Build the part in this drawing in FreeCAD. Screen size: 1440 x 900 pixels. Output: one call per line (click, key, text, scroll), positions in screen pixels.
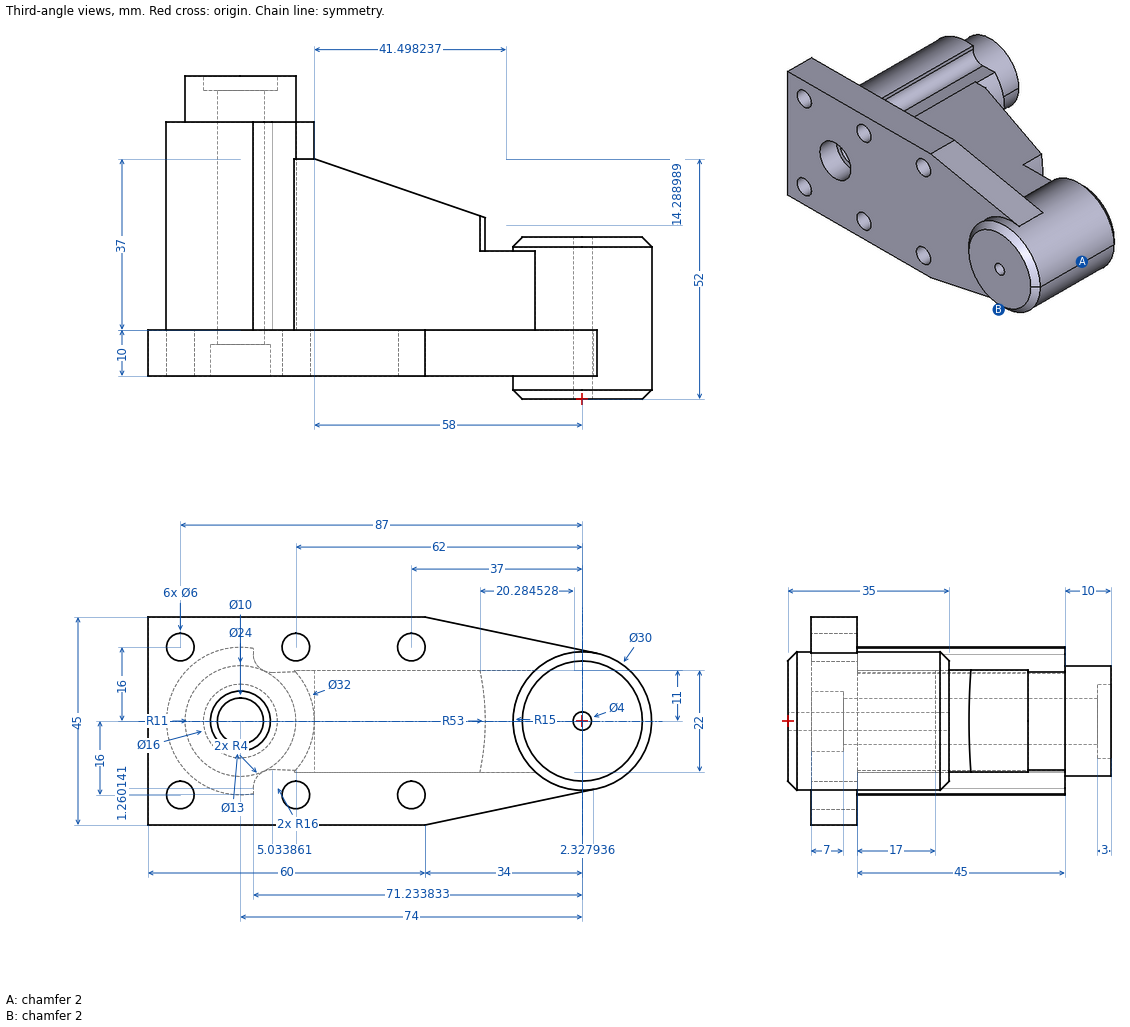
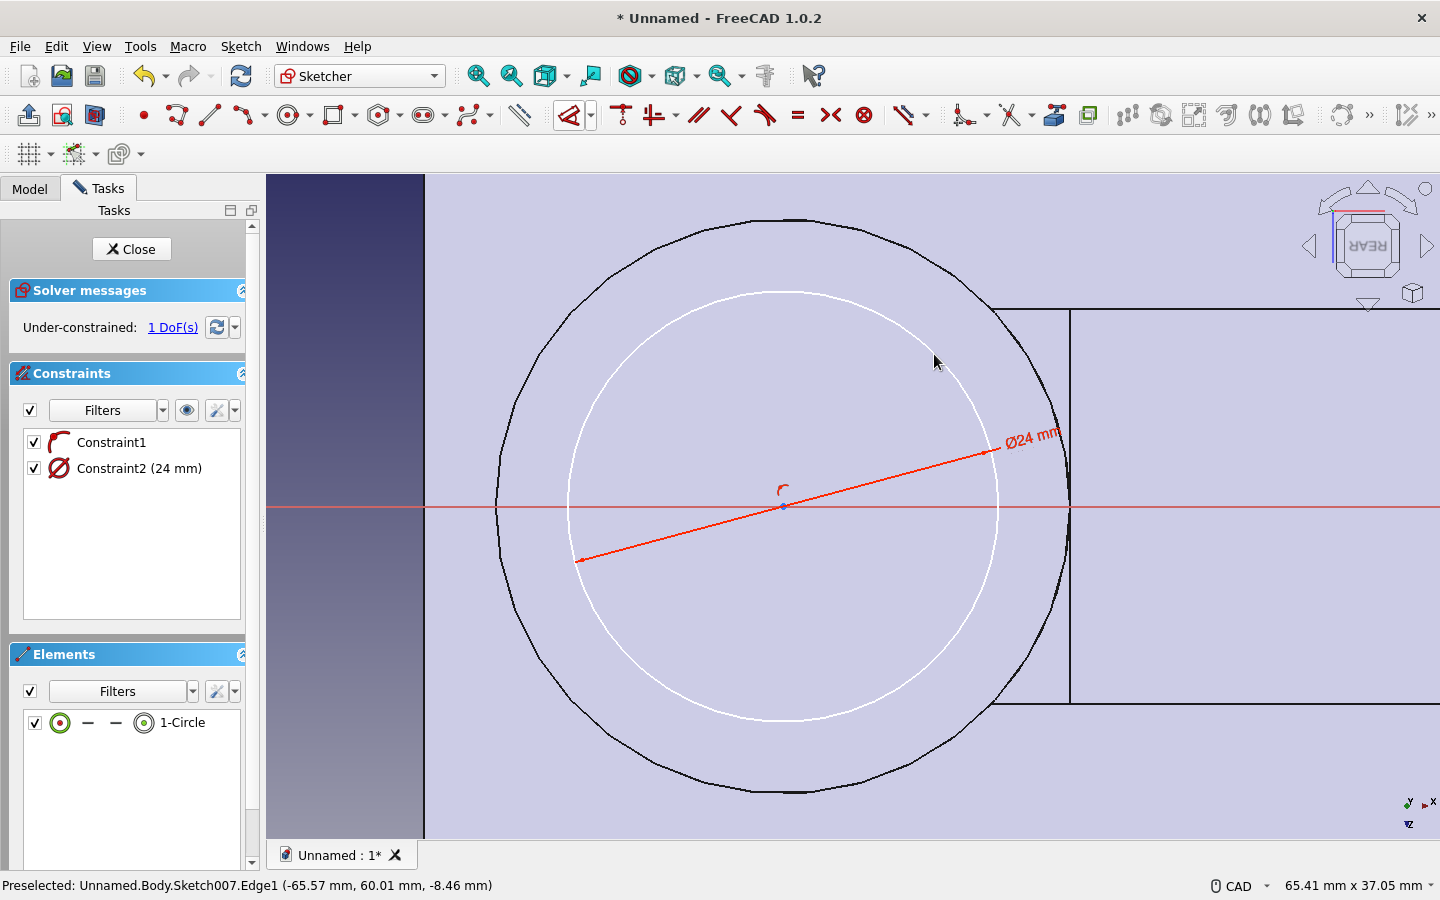
click(783, 506)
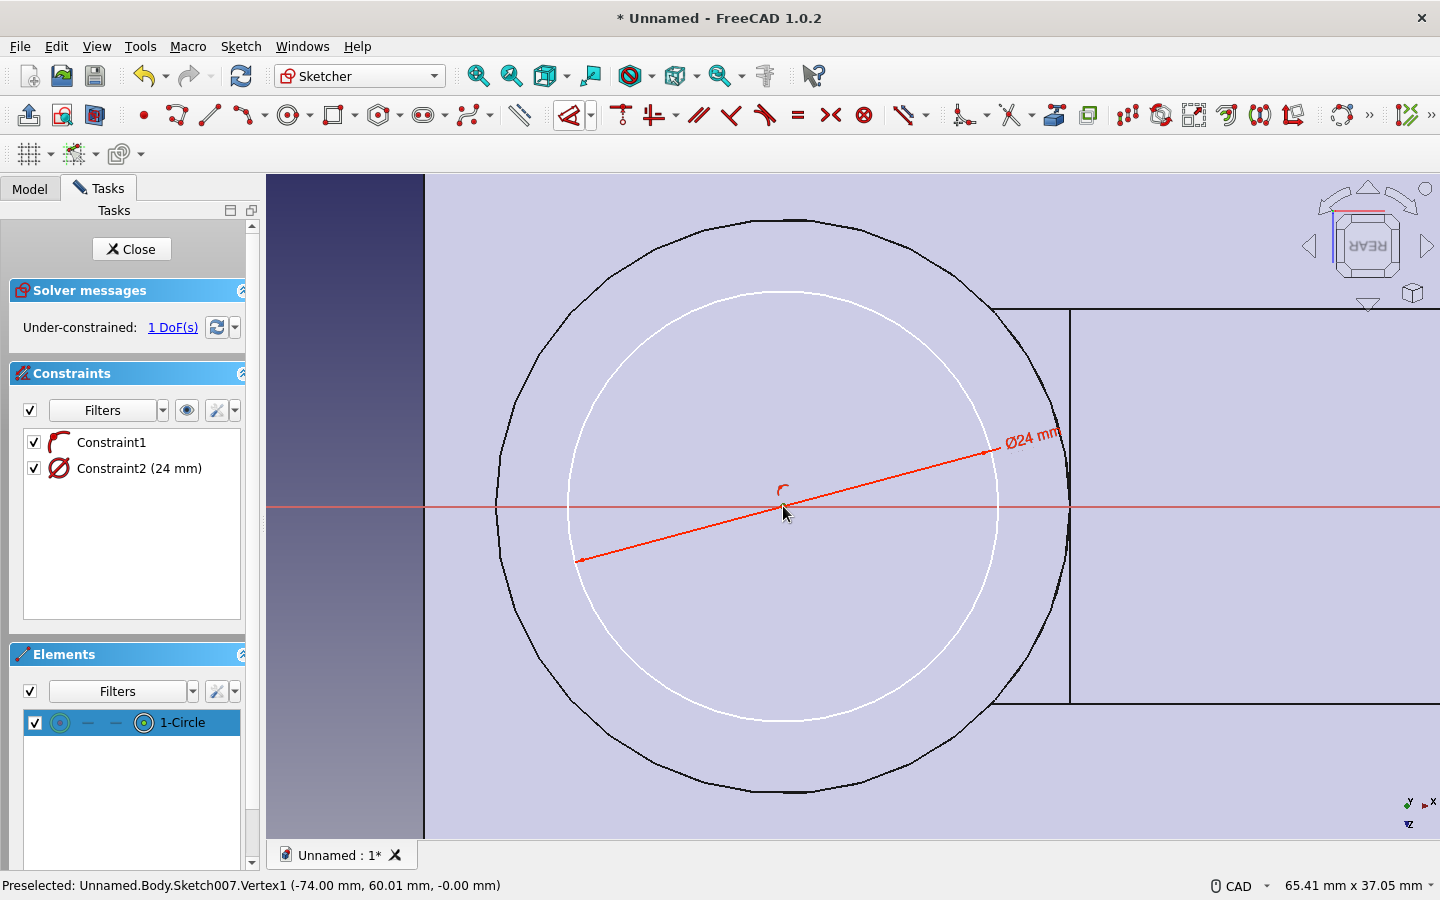
click(590, 116)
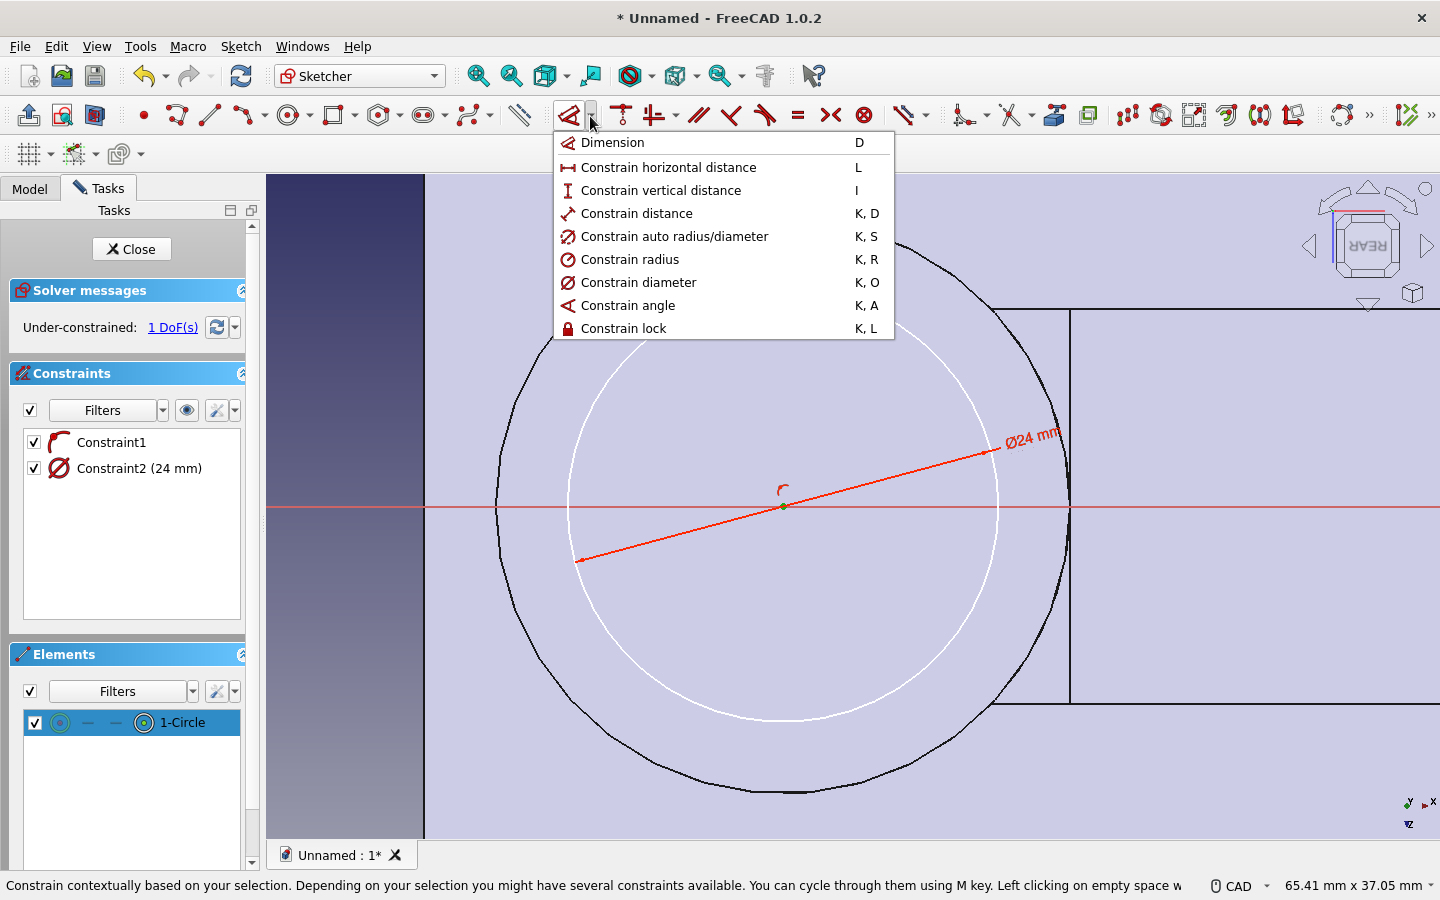
click(724, 168)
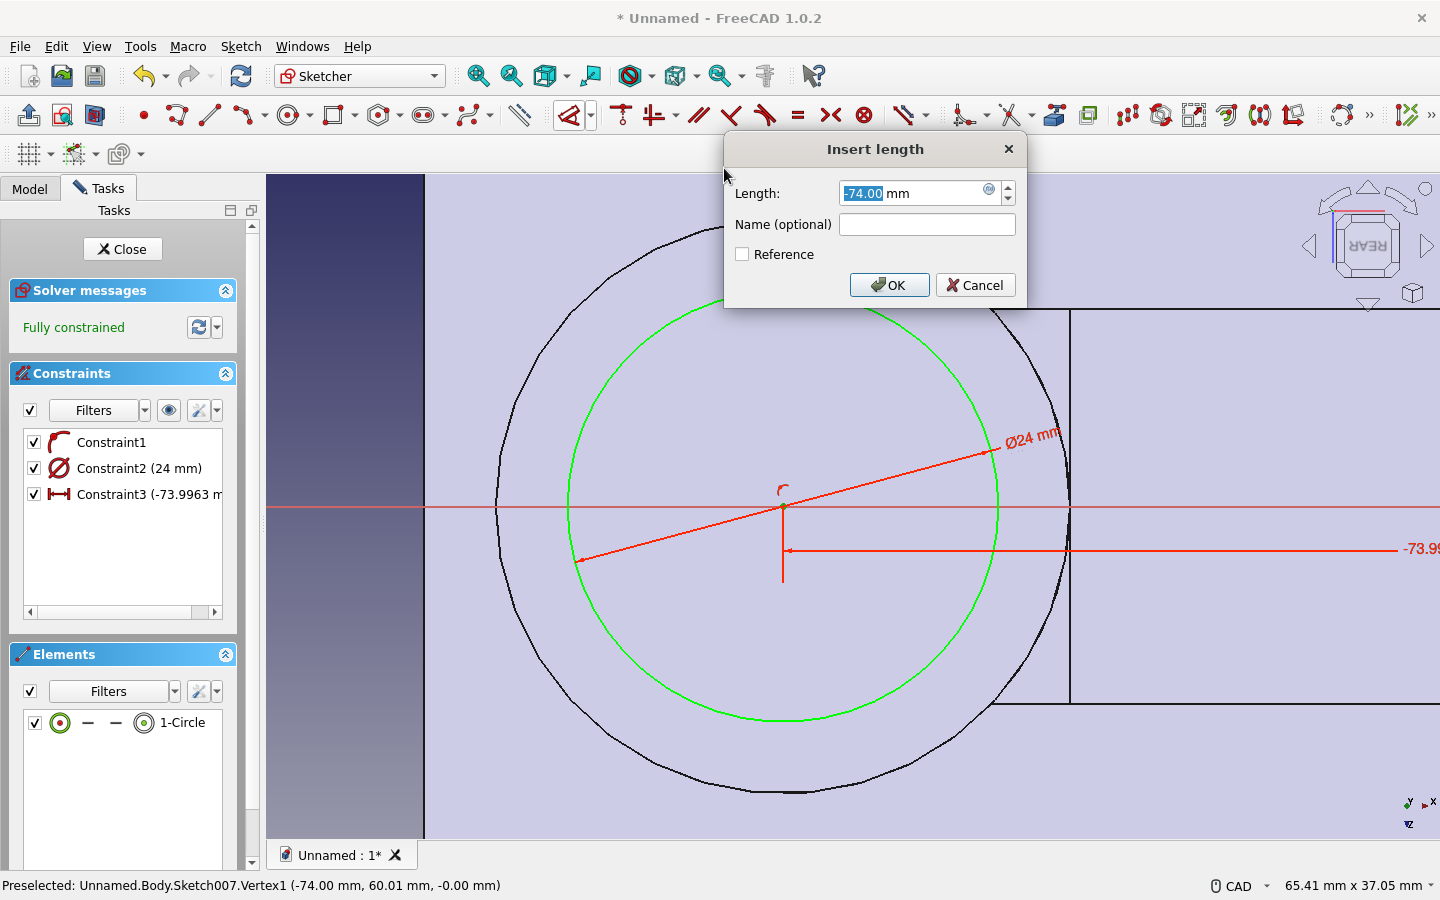
text(-74)
key(Return)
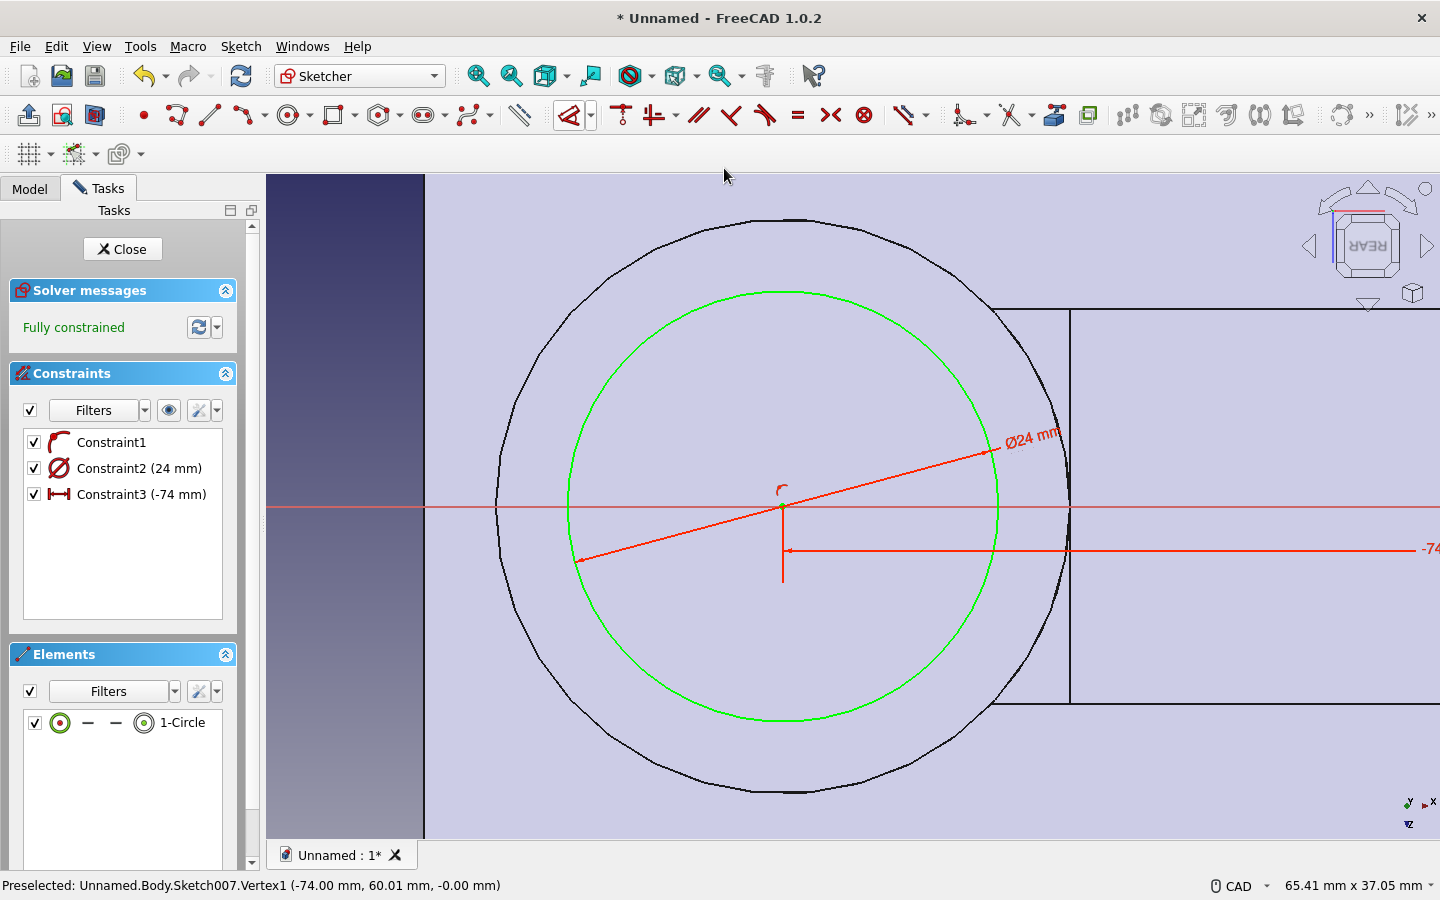
click(123, 249)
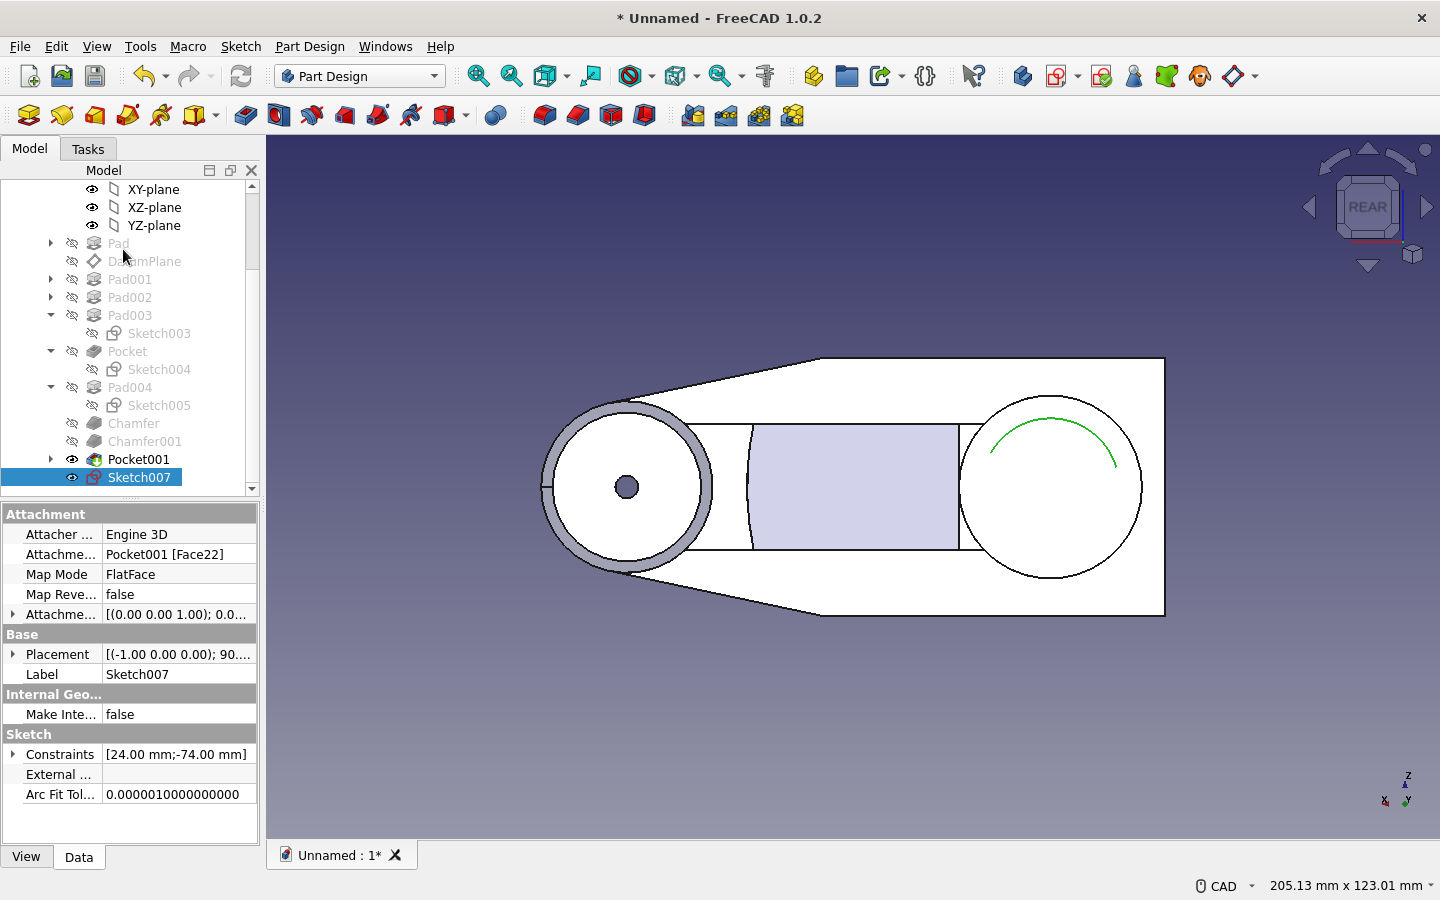
click(29, 116)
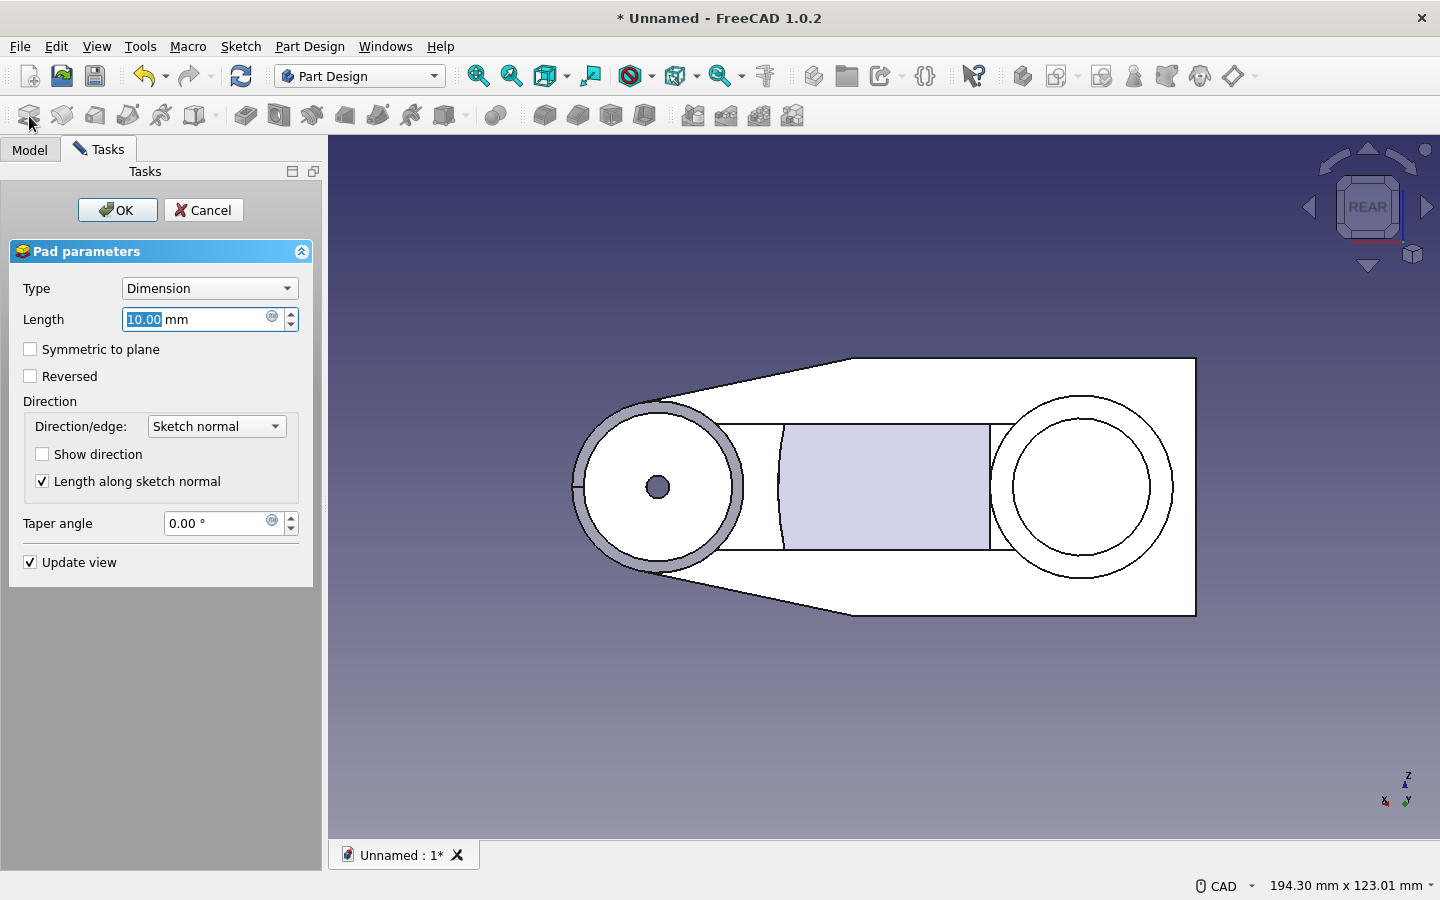
text(10)
key(Tab)